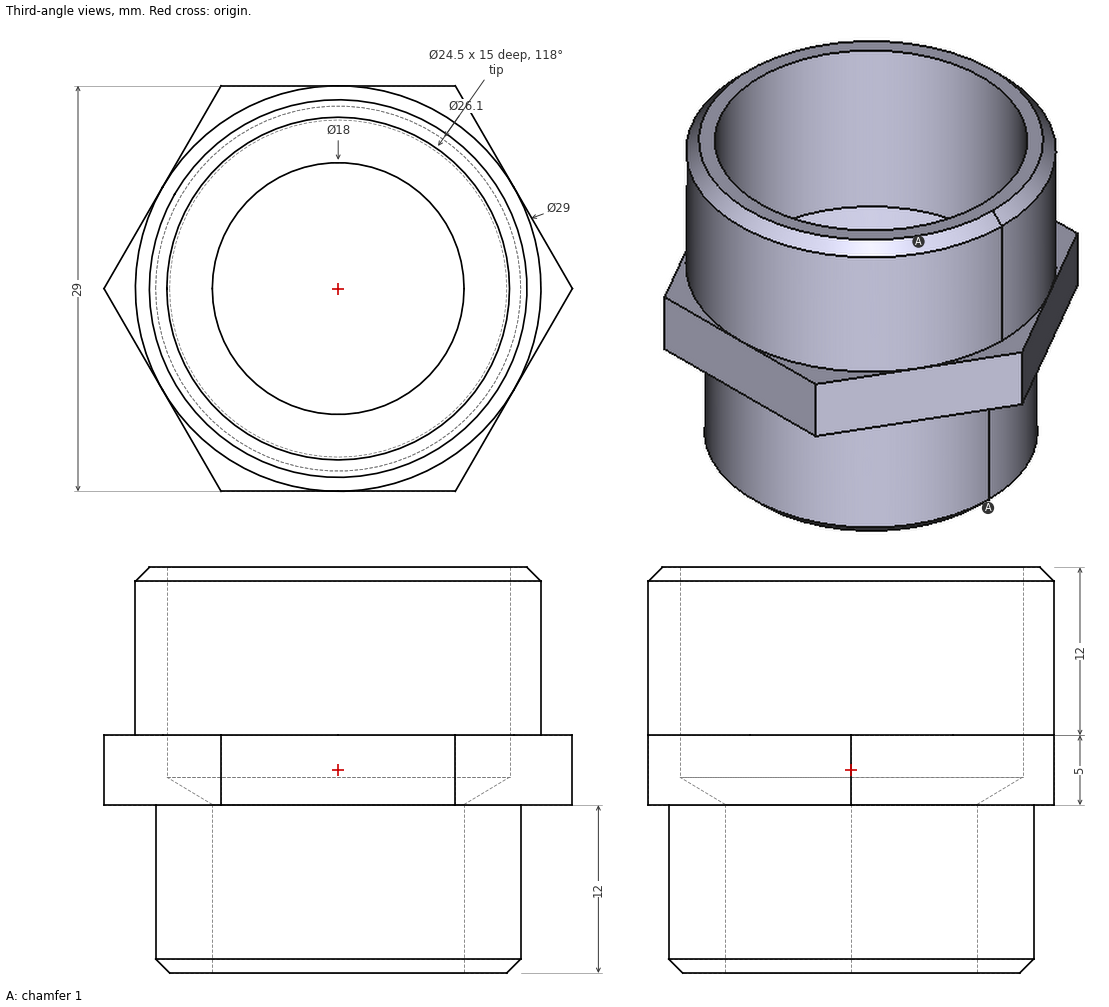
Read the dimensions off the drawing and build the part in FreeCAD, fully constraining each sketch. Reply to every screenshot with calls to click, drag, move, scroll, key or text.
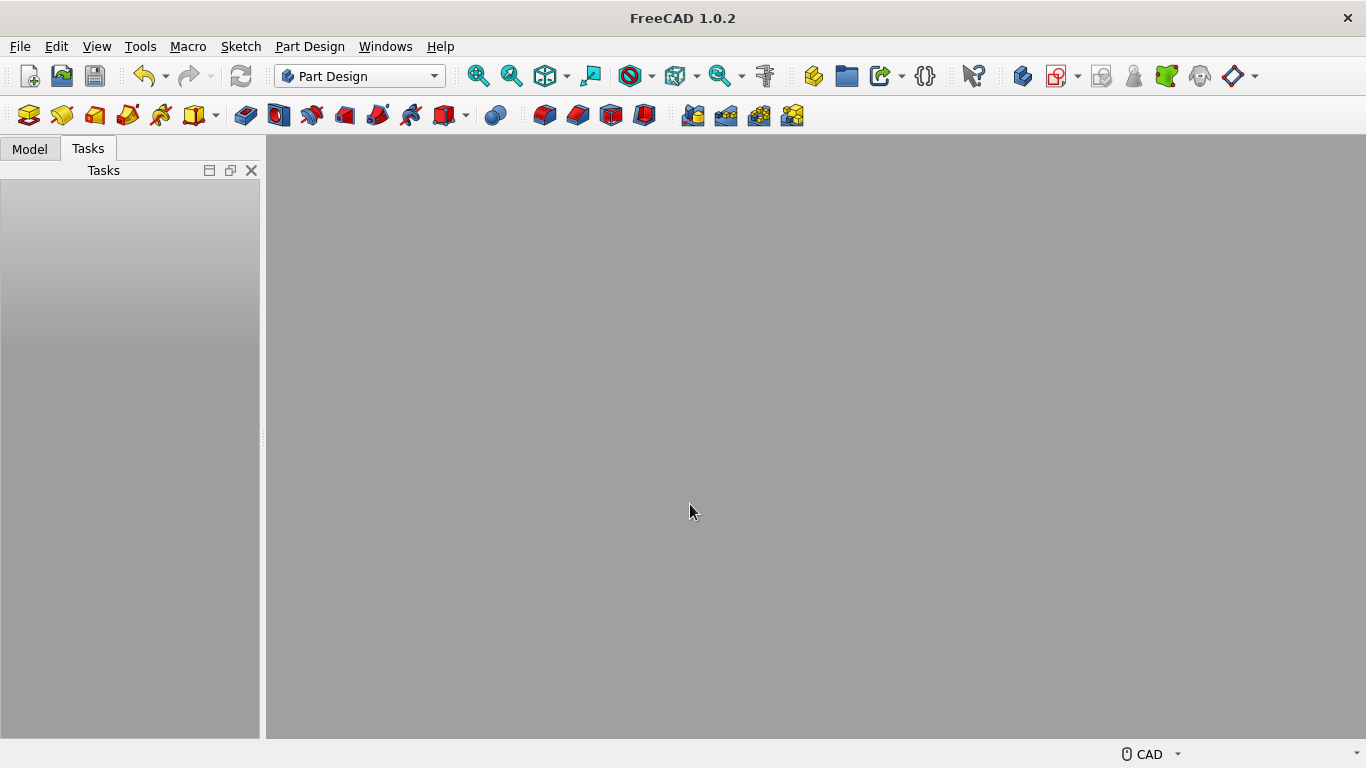
click(29, 76)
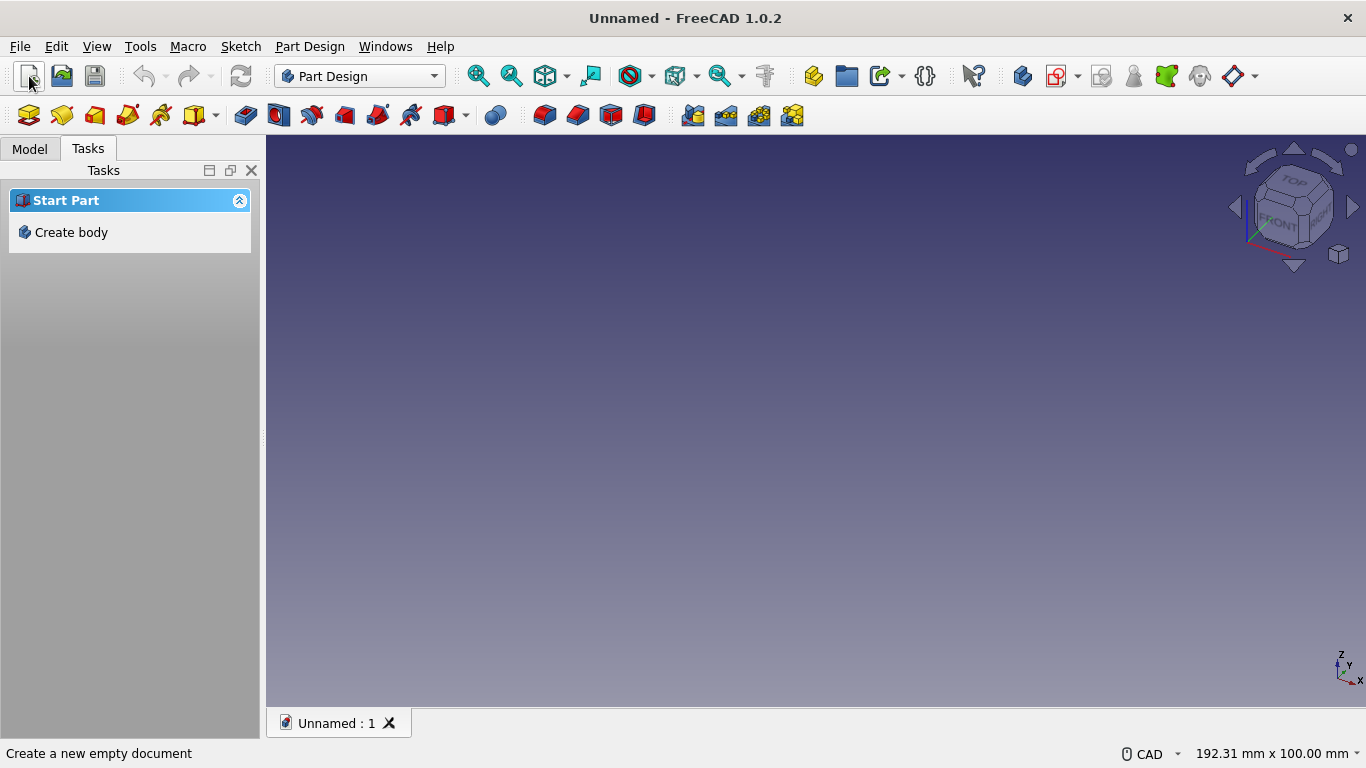
click(1056, 76)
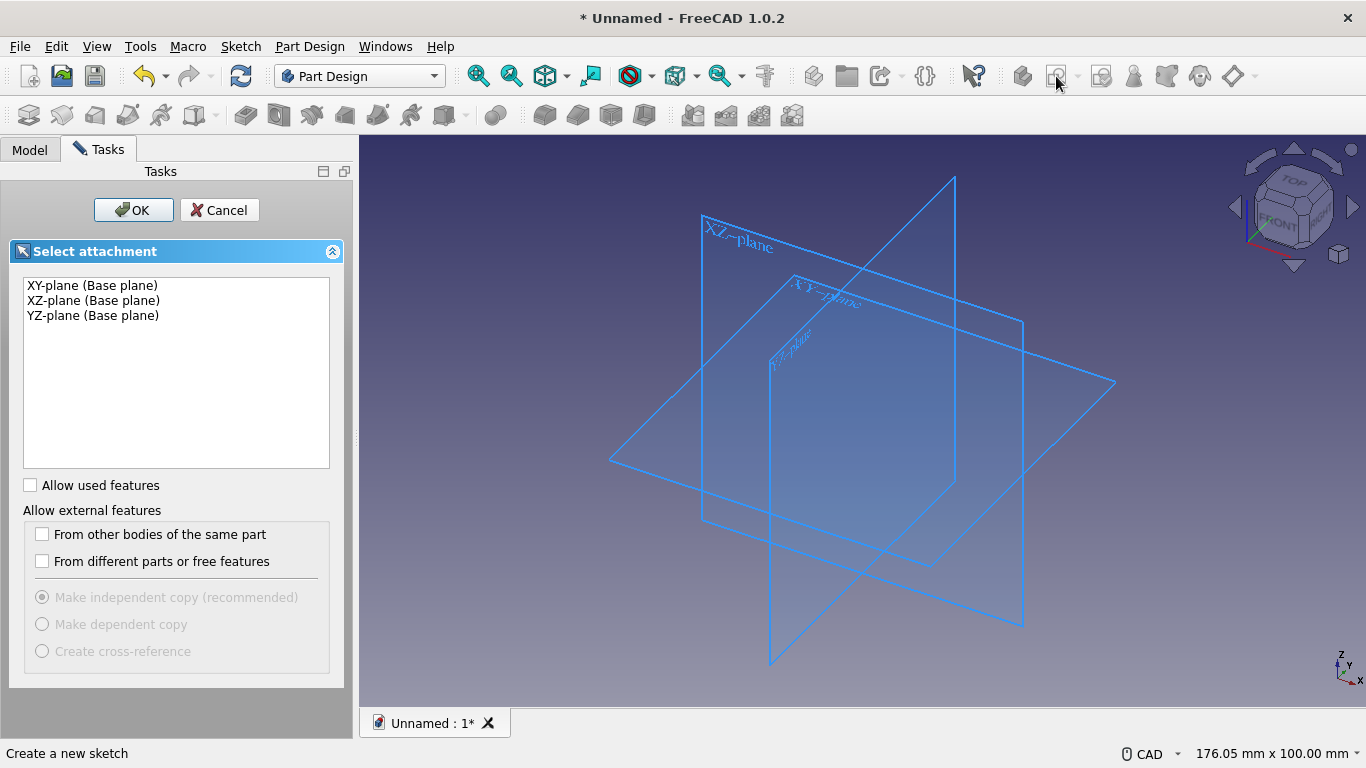
click(84, 286)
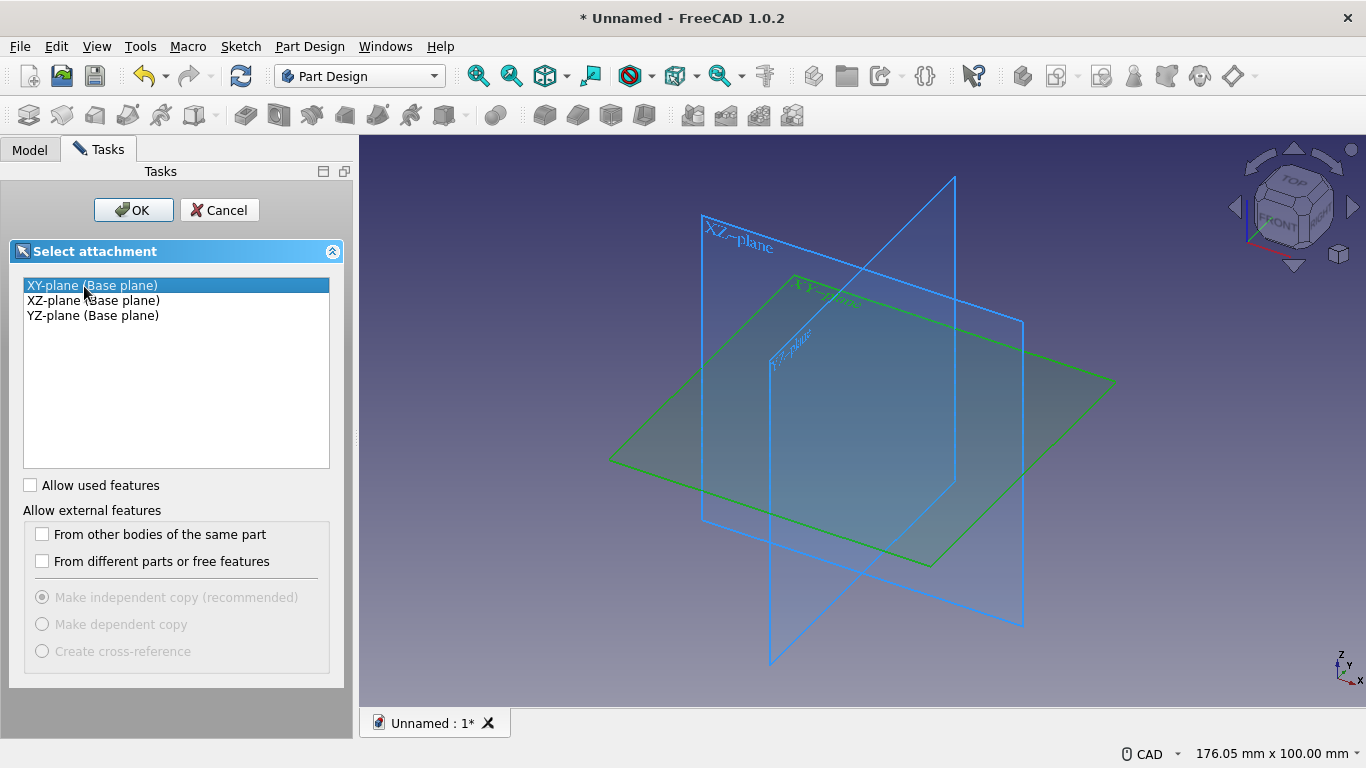
click(134, 210)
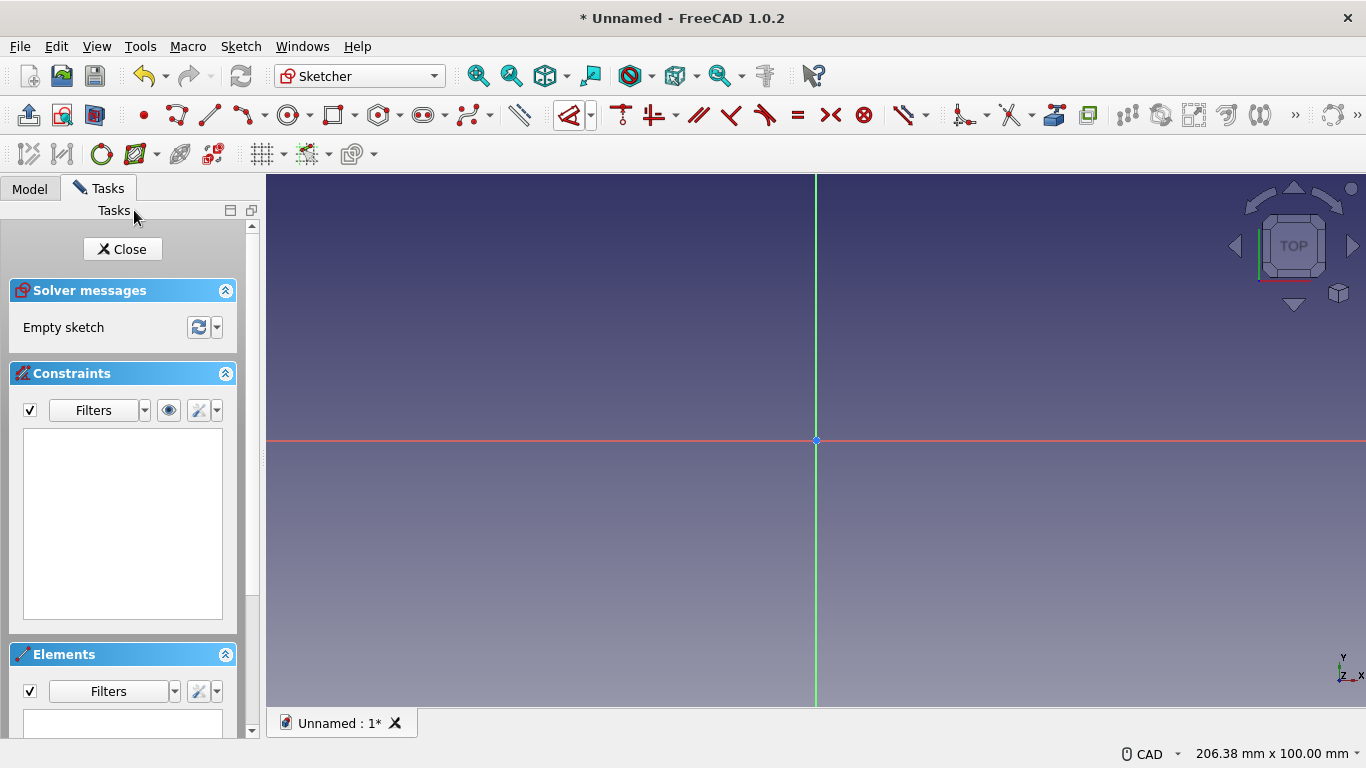
scroll(872, 440, up, 4)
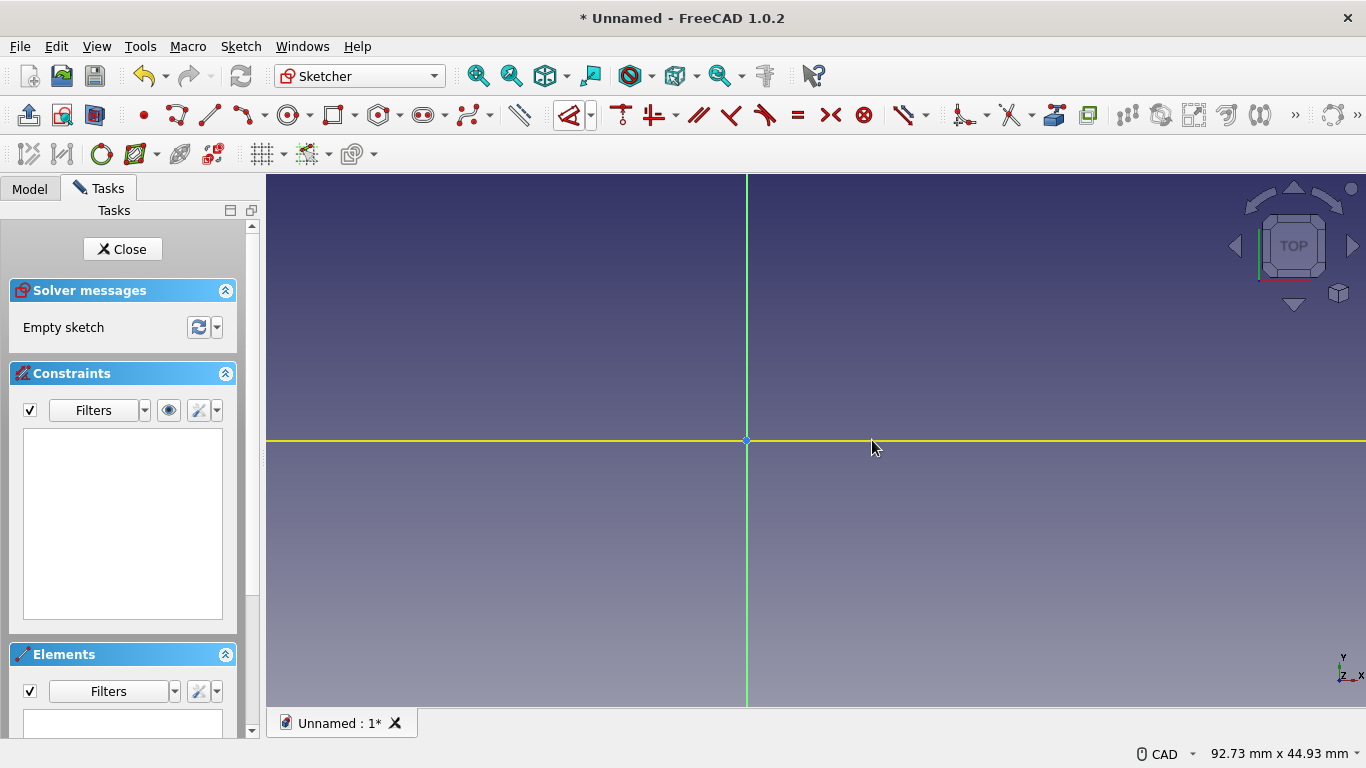
click(378, 116)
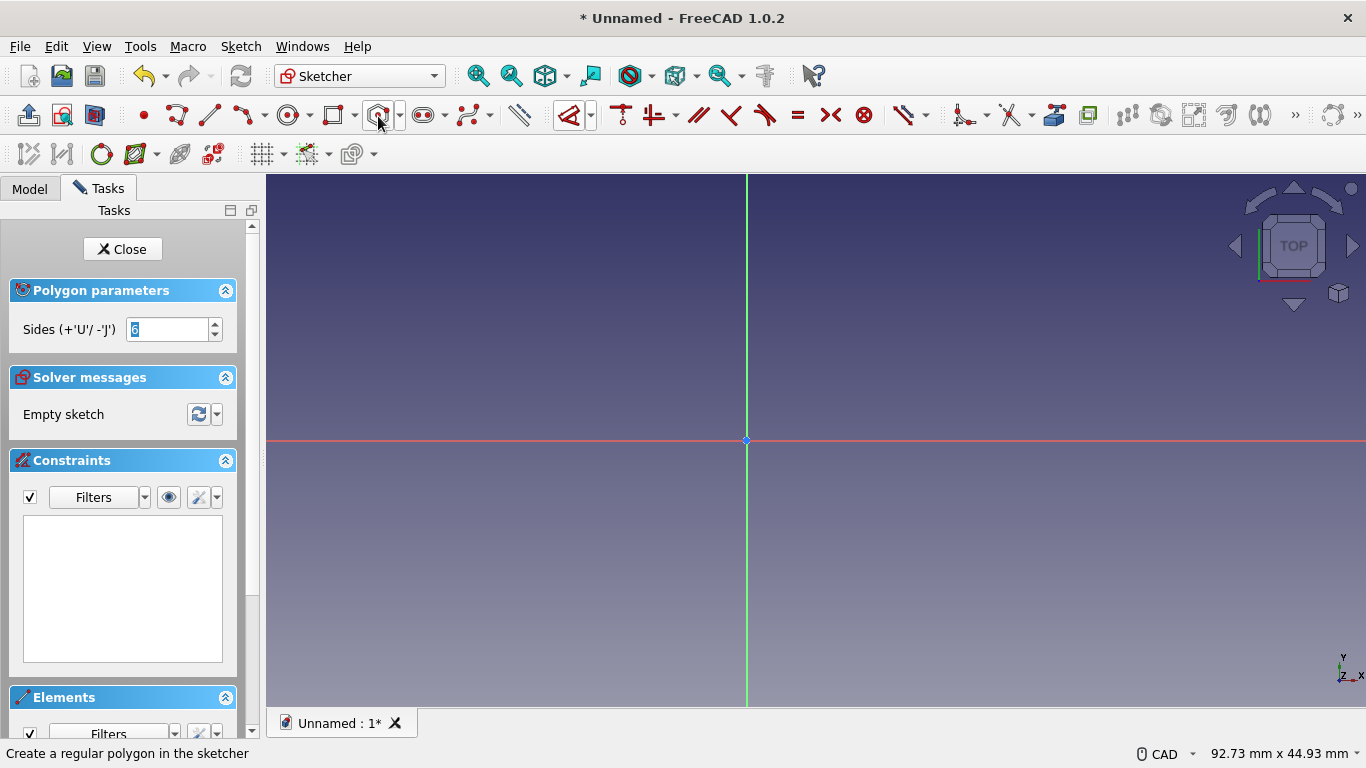
click(747, 440)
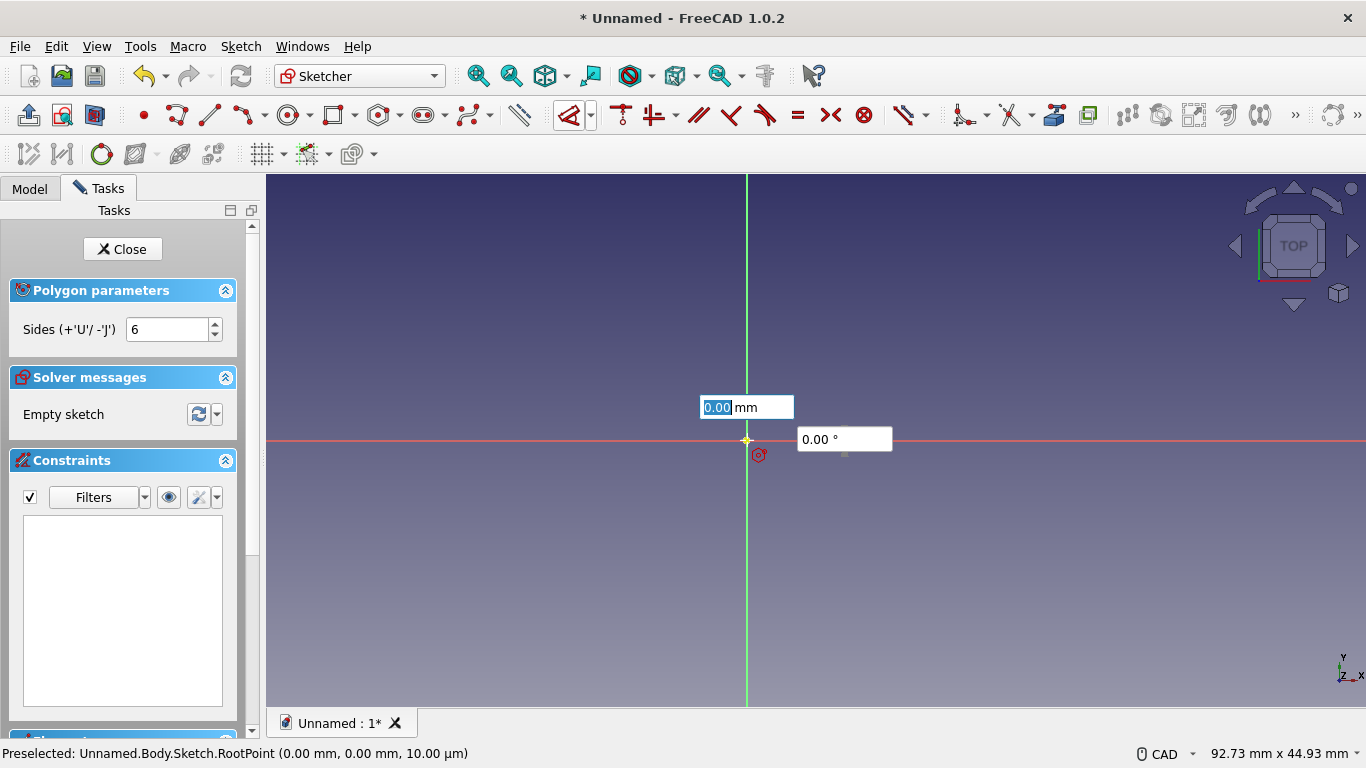
click(945, 440)
right_click(945, 440)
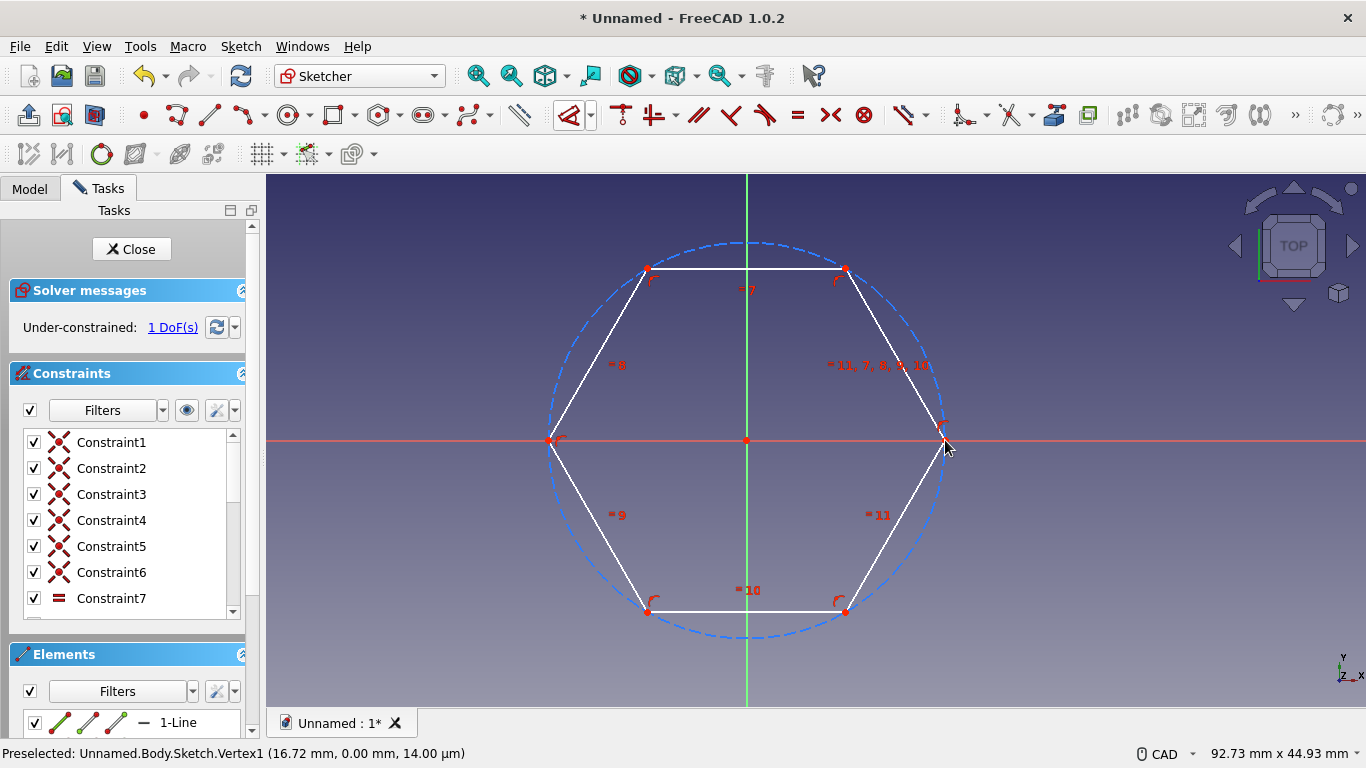
click(568, 116)